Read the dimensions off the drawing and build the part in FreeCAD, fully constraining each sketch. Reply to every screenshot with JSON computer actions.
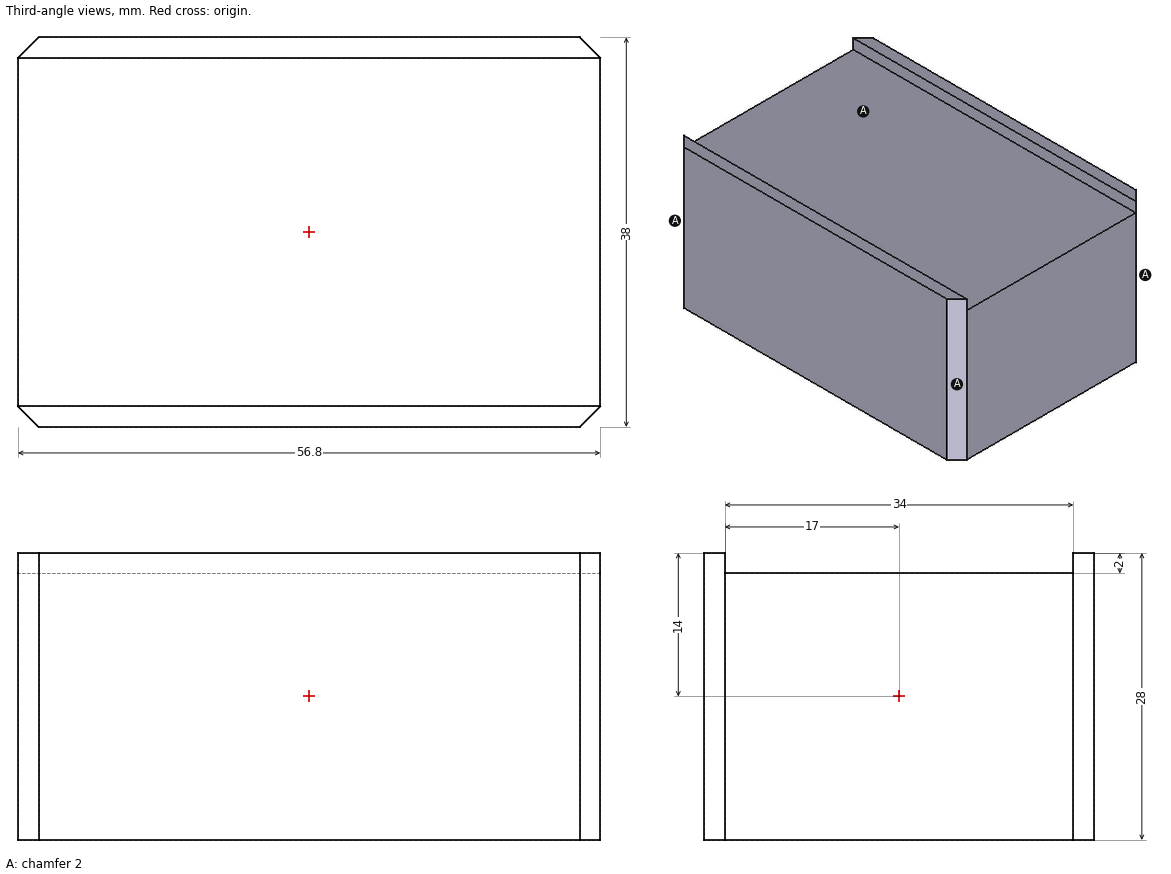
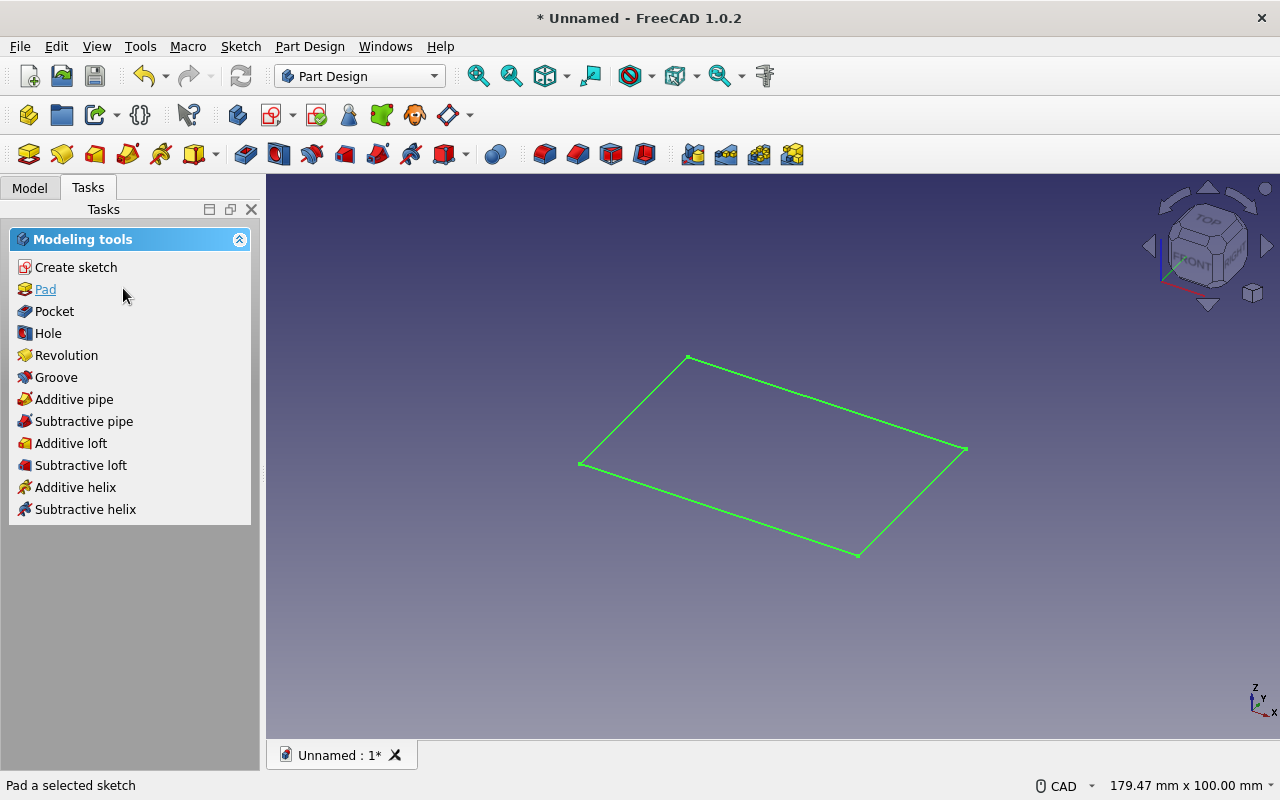
{"action": "left_click", "coordinate": [29, 154]}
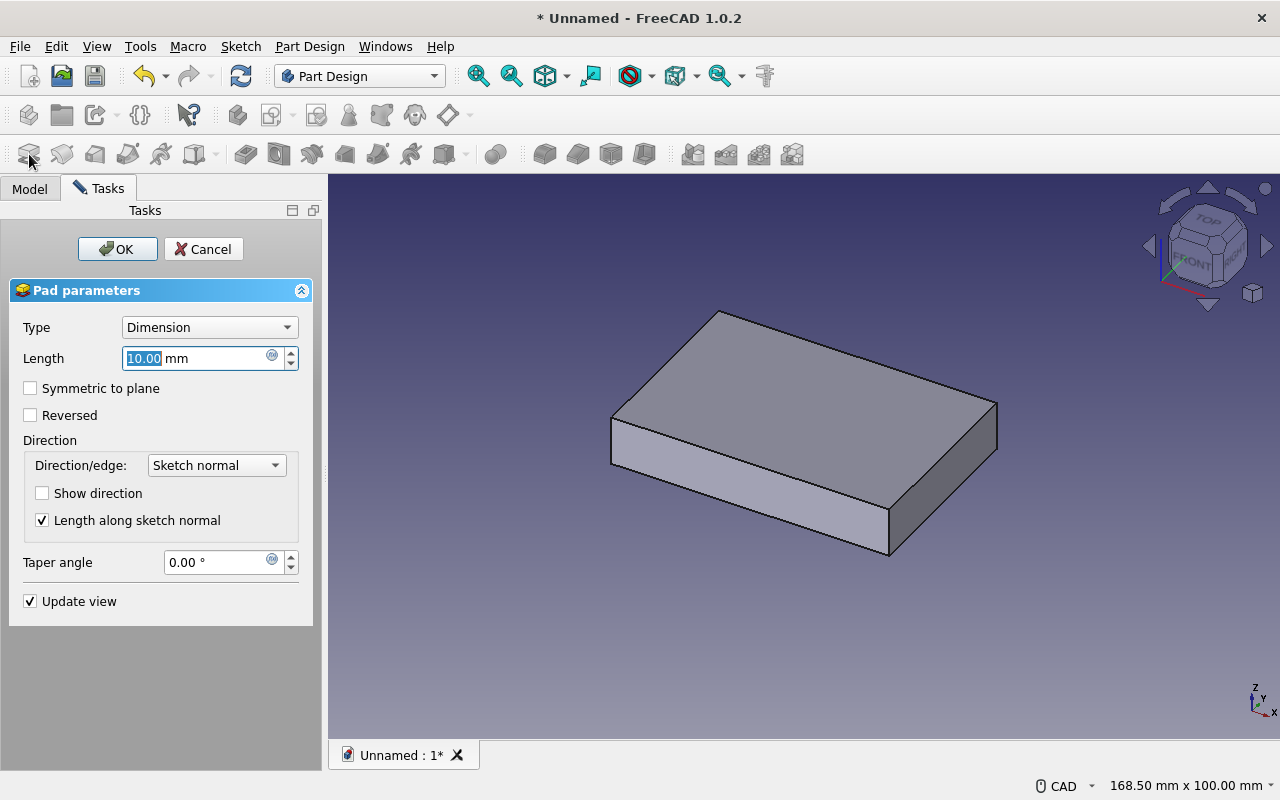
{"action": "type", "text": "28"}
{"action": "key", "text": "Tab"}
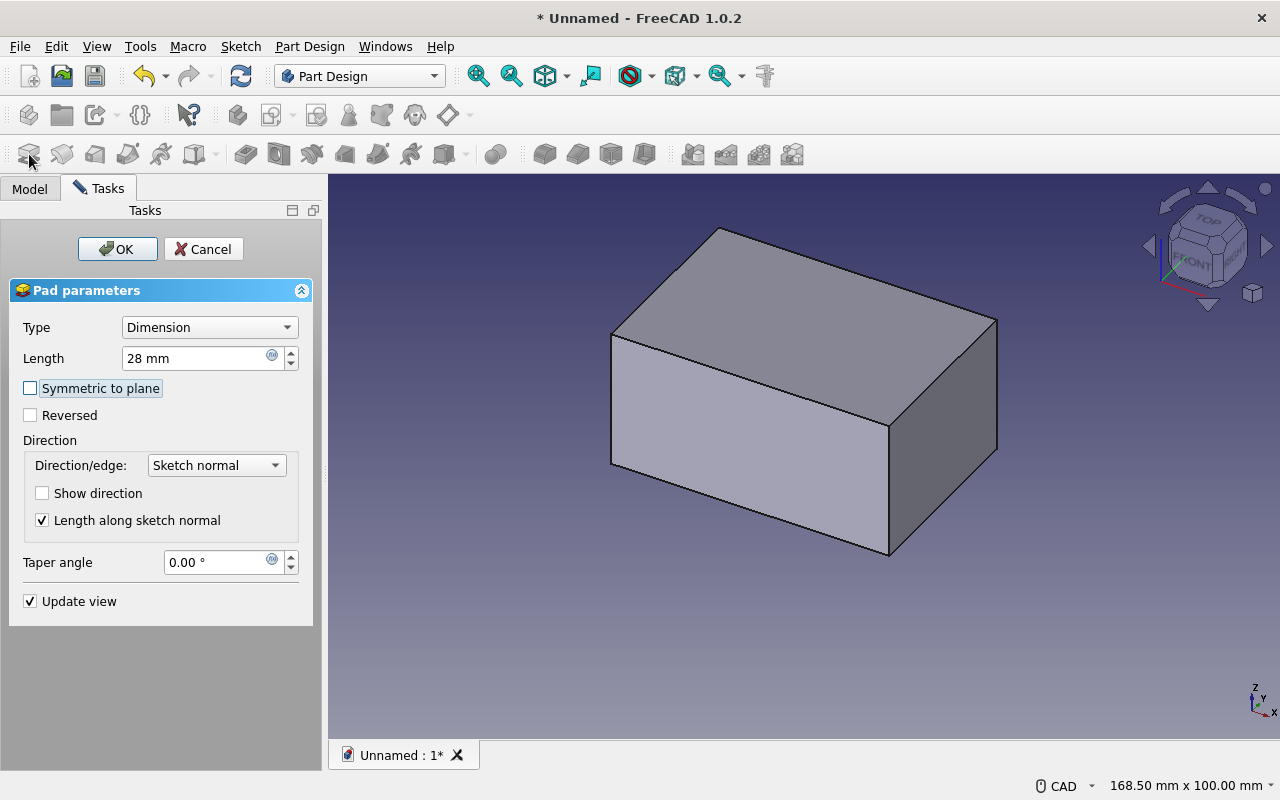
{"action": "left_click", "coordinate": [31, 388]}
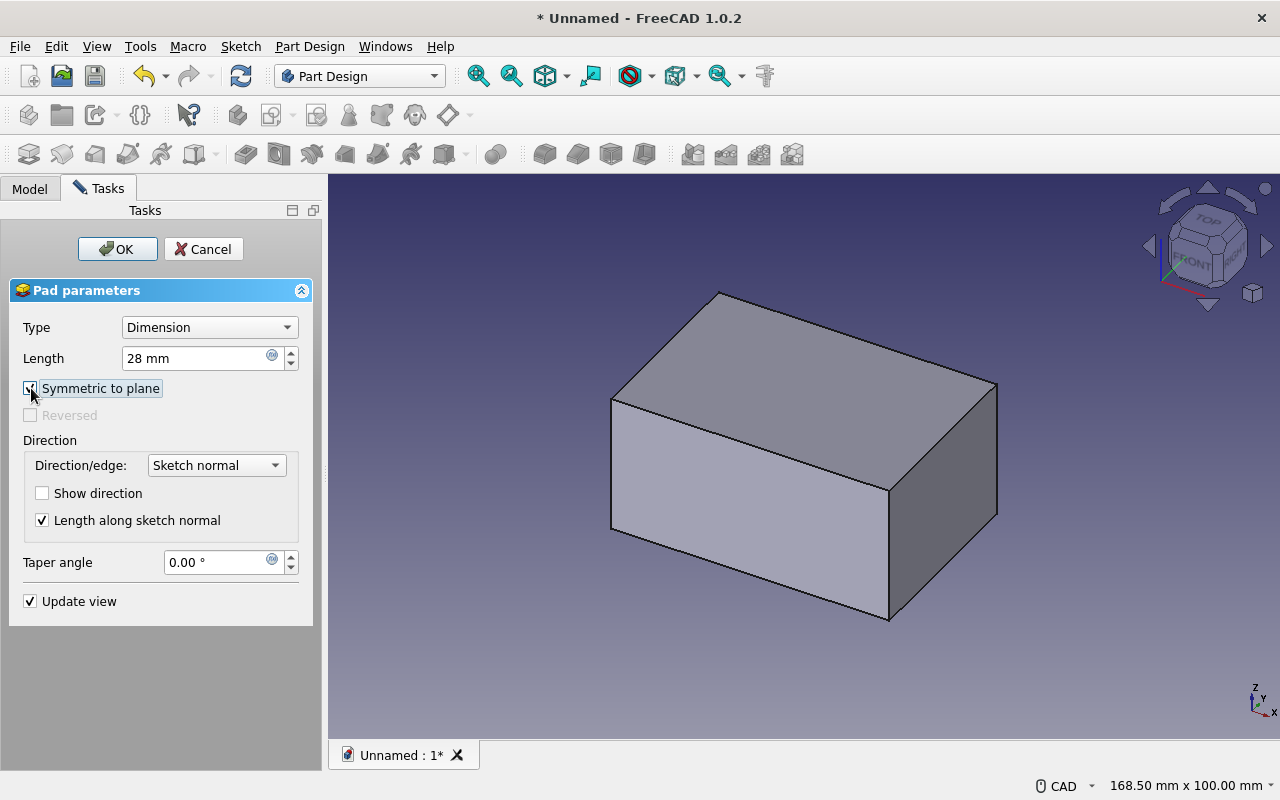
{"action": "left_click", "coordinate": [118, 249]}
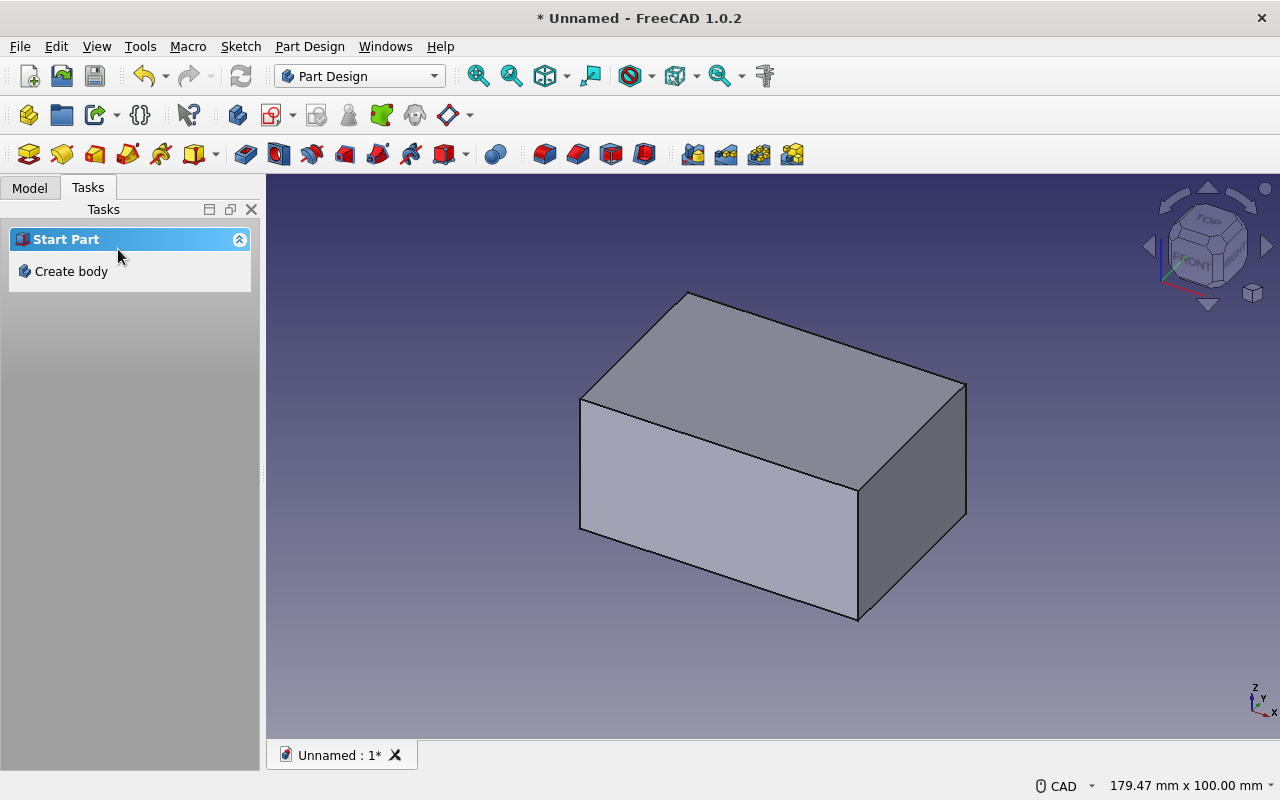
{"action": "left_click", "coordinate": [858, 555]}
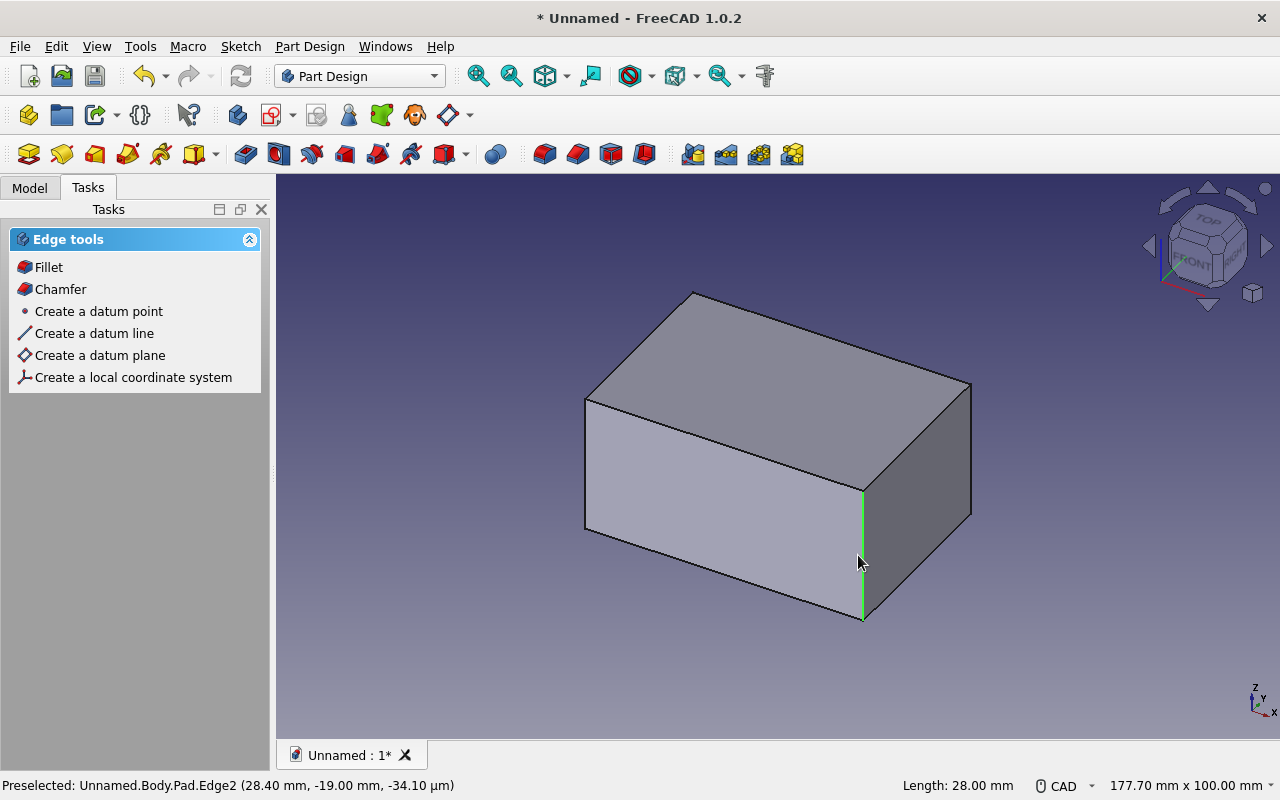
{"action": "key", "text": "0"}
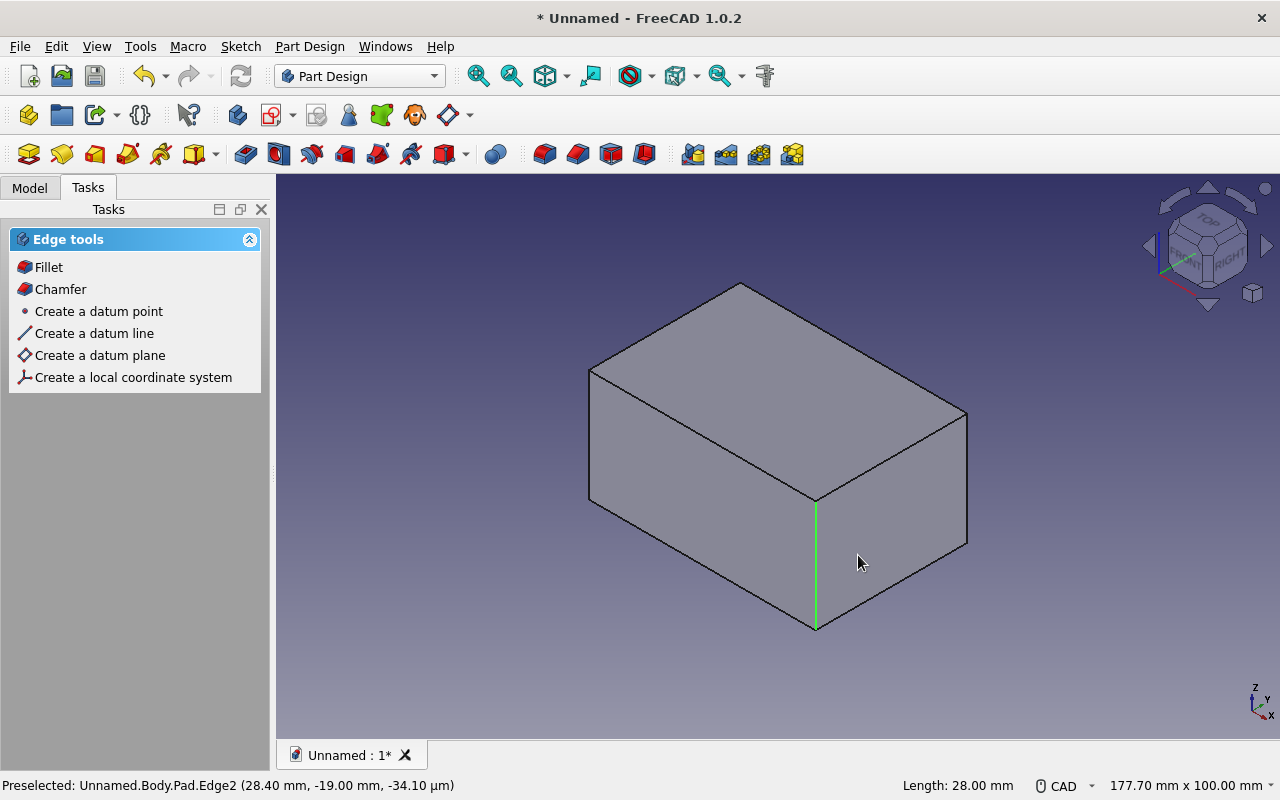
{"action": "key", "text": "2"}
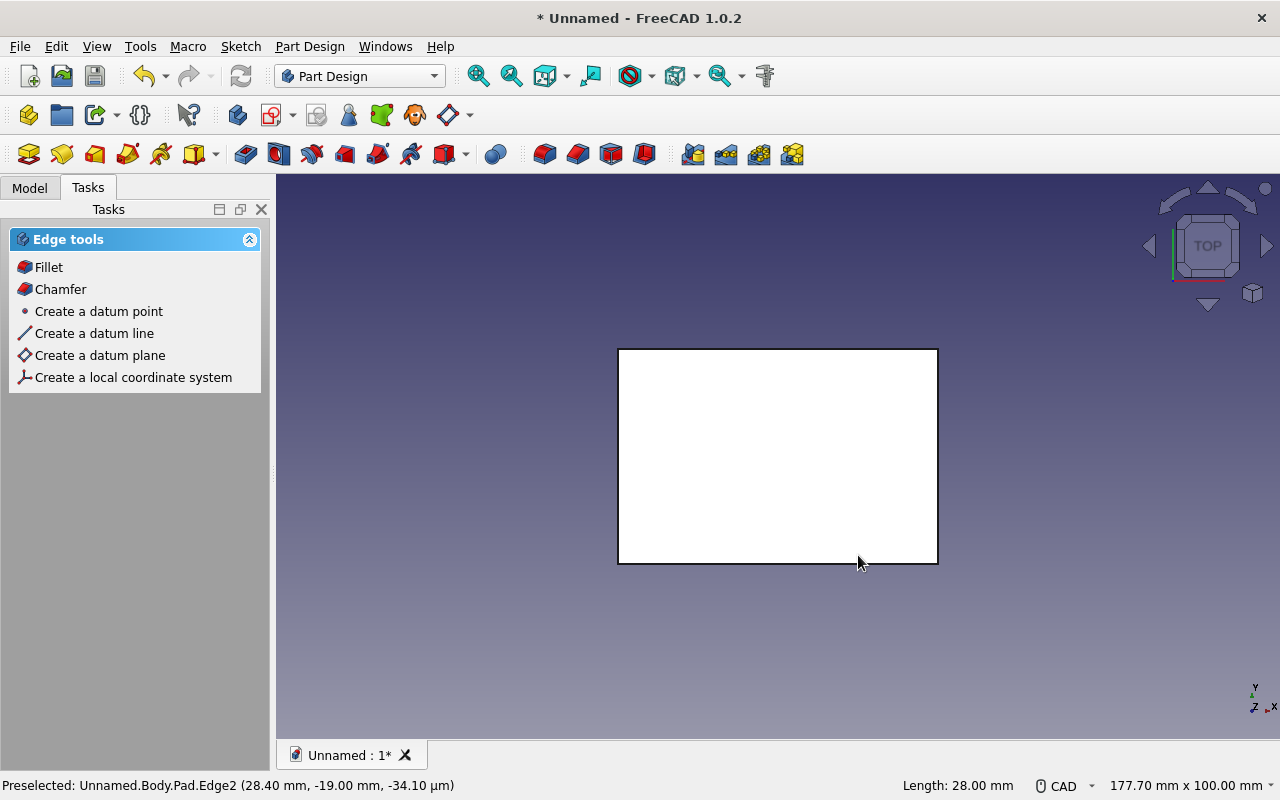
{"action": "left_click", "coordinate": [479, 76]}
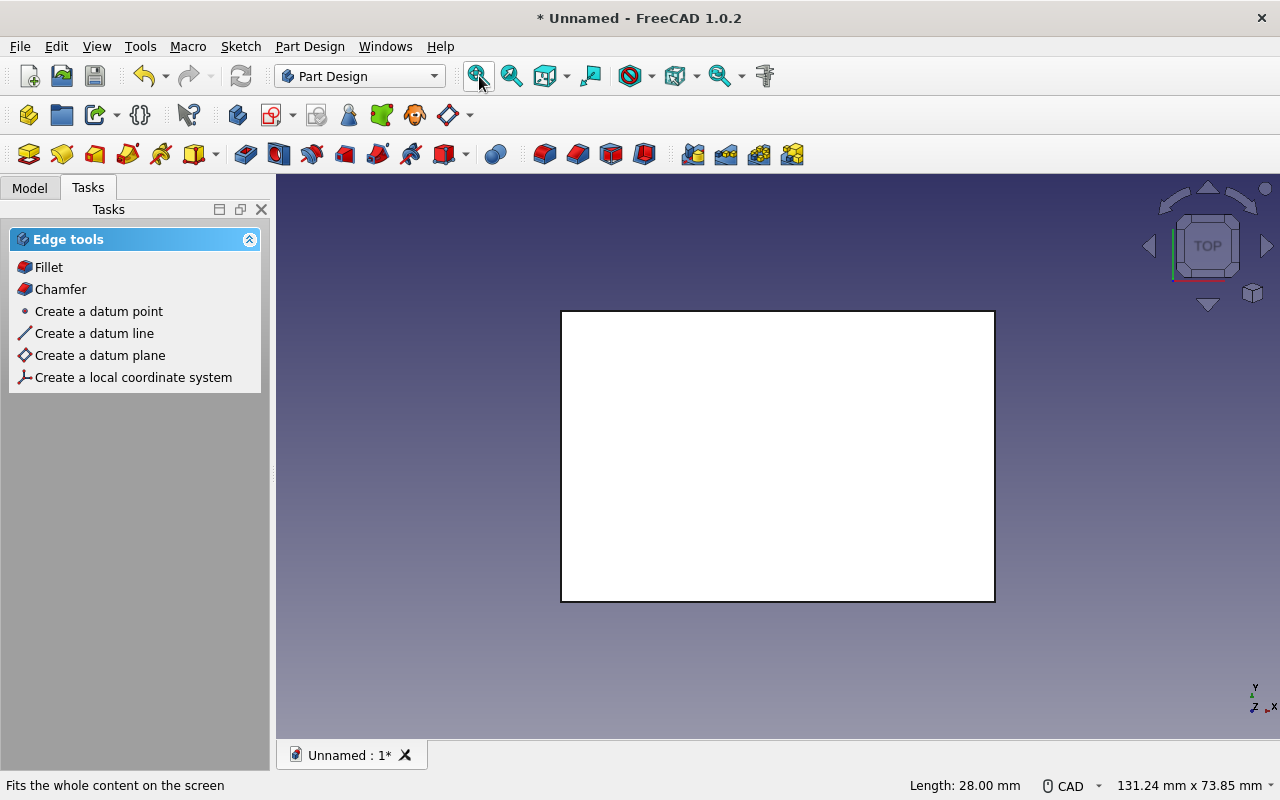
{"action": "key", "text": "1"}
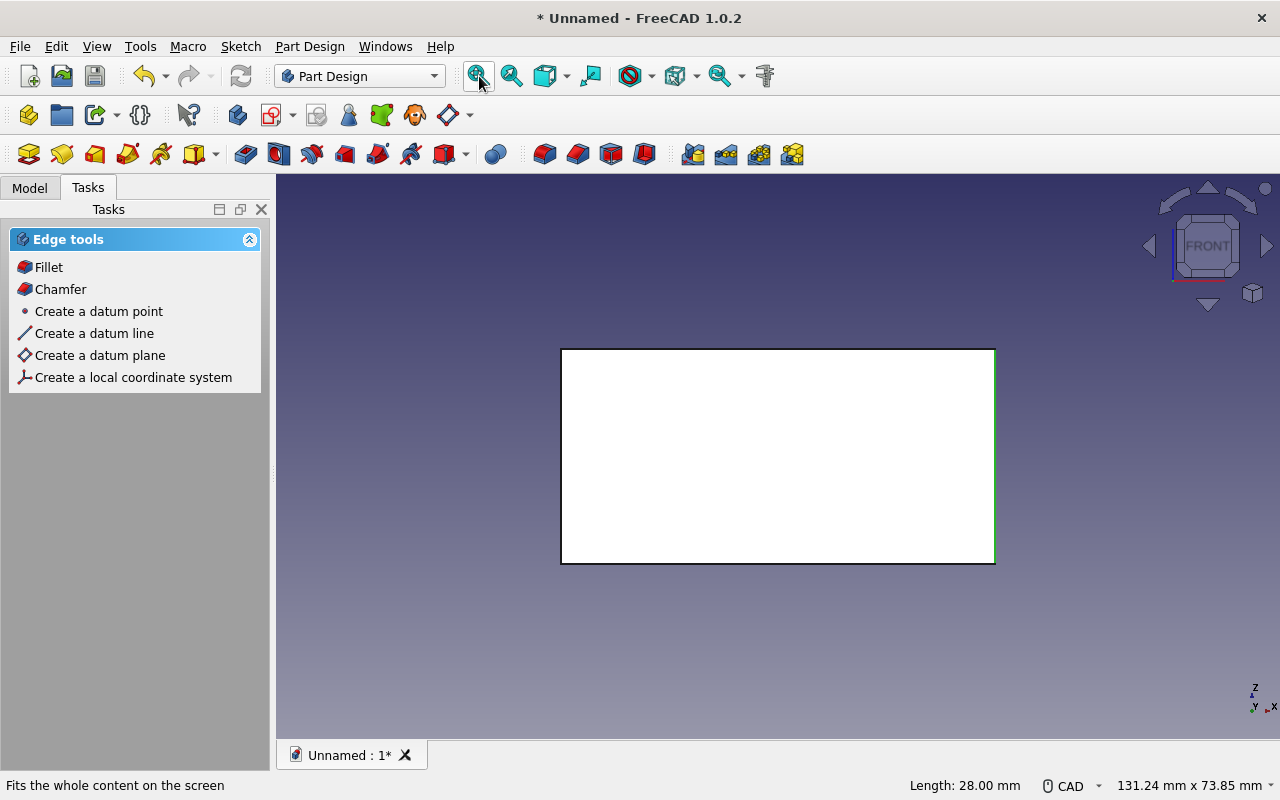
{"action": "left_click", "coordinate": [479, 76]}